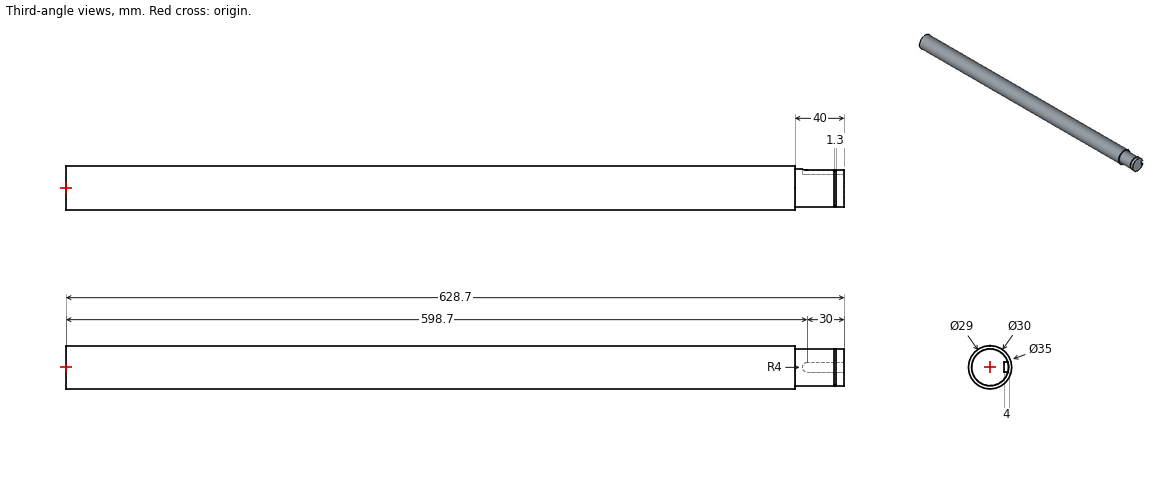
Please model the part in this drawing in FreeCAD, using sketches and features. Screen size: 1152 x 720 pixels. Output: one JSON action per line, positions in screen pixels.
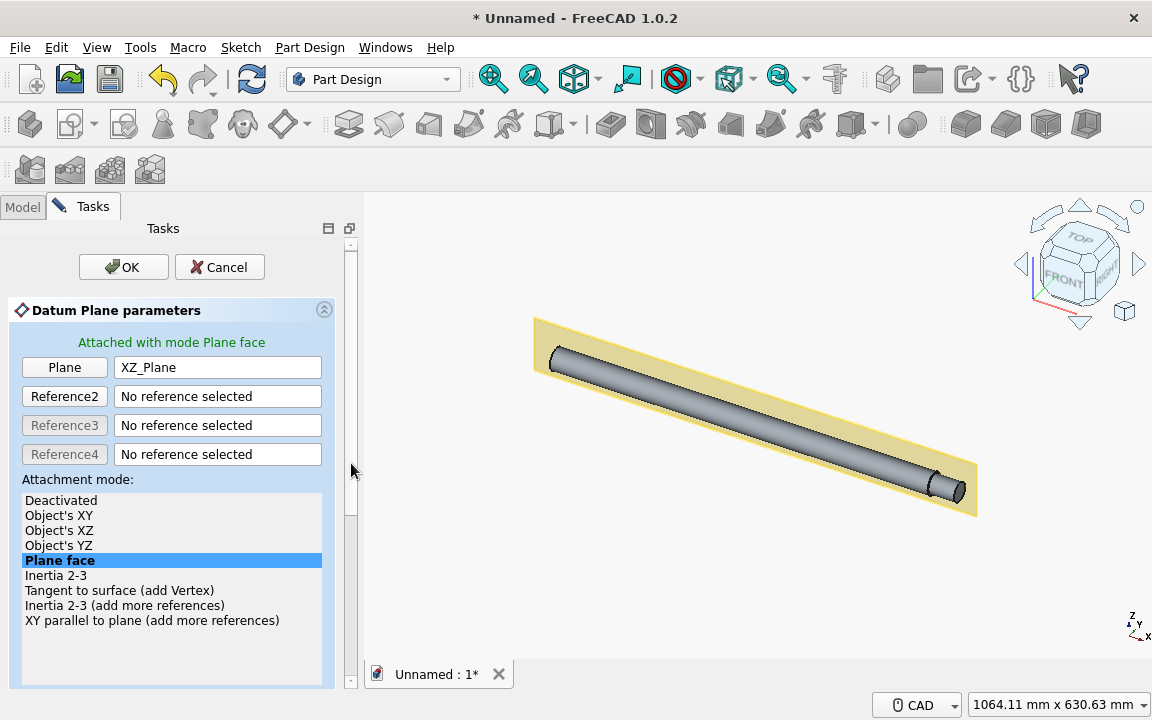
{"action": "left_click", "coordinate": [124, 267]}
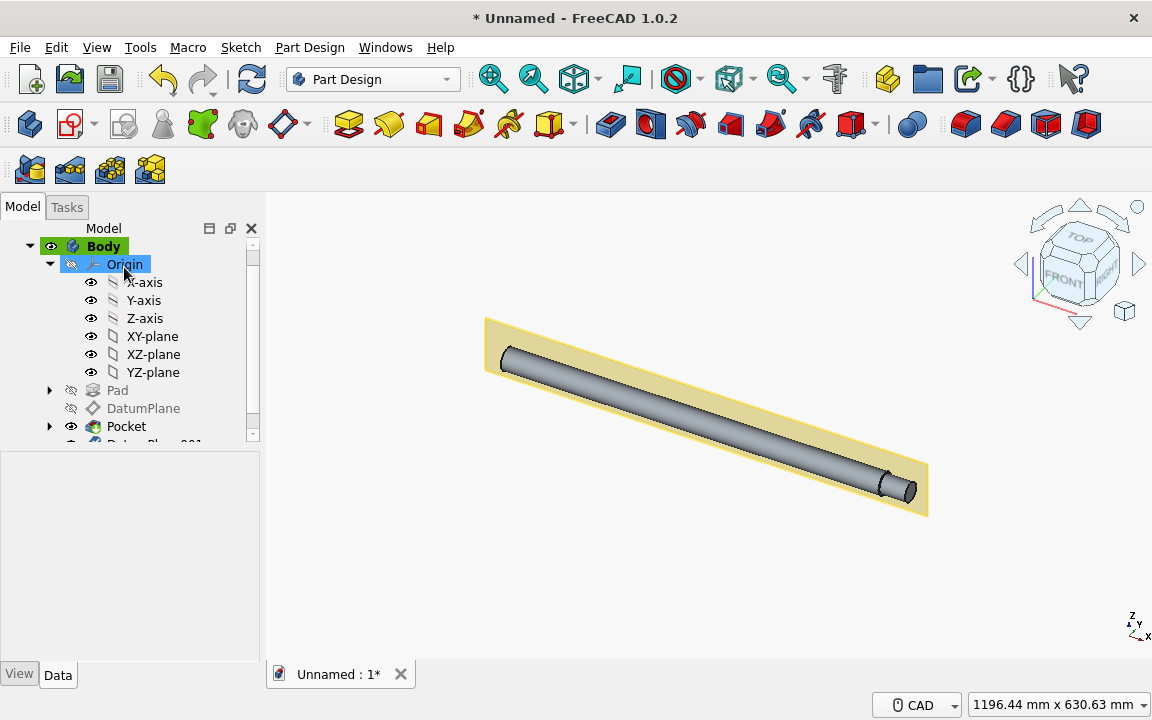
{"action": "scroll", "coordinate": [120, 332], "scroll_direction": "down", "scroll_amount": 3}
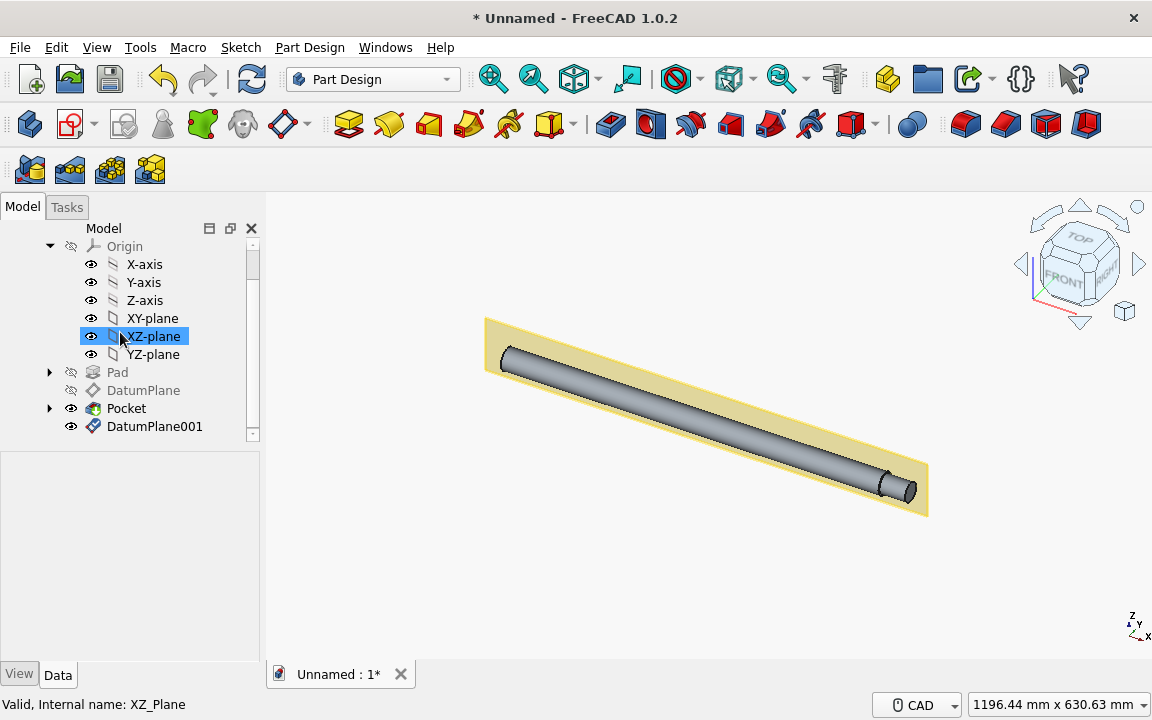
{"action": "left_click", "coordinate": [116, 426]}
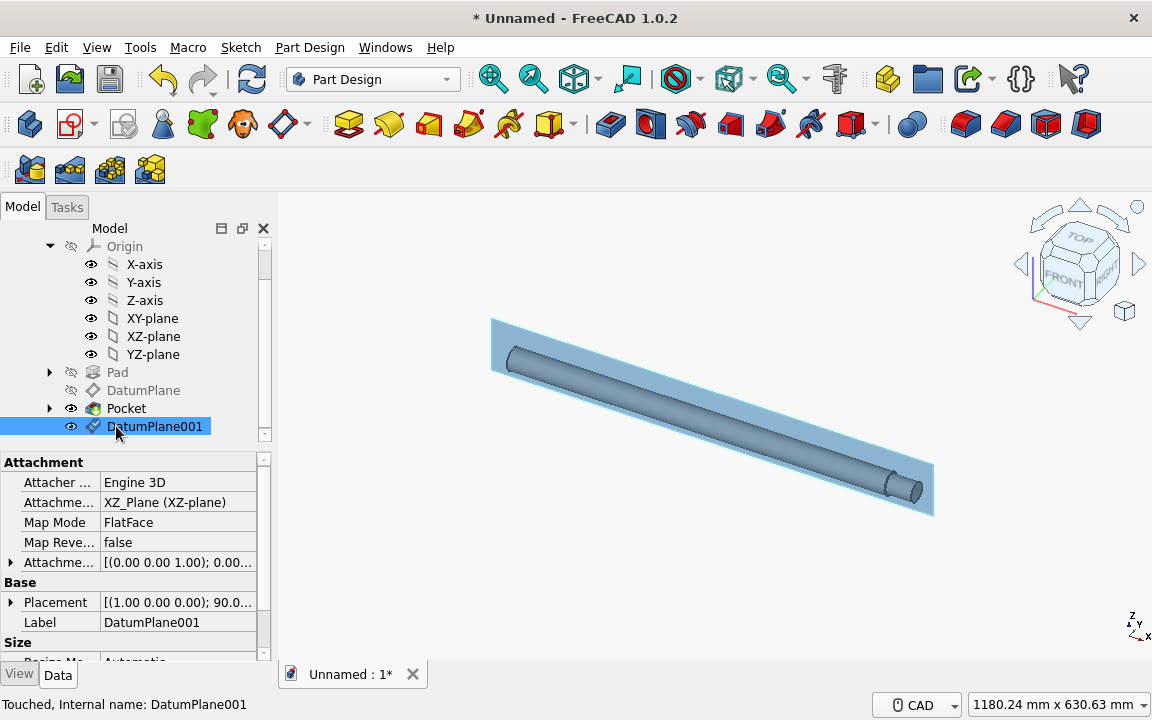
{"action": "left_click", "coordinate": [70, 124]}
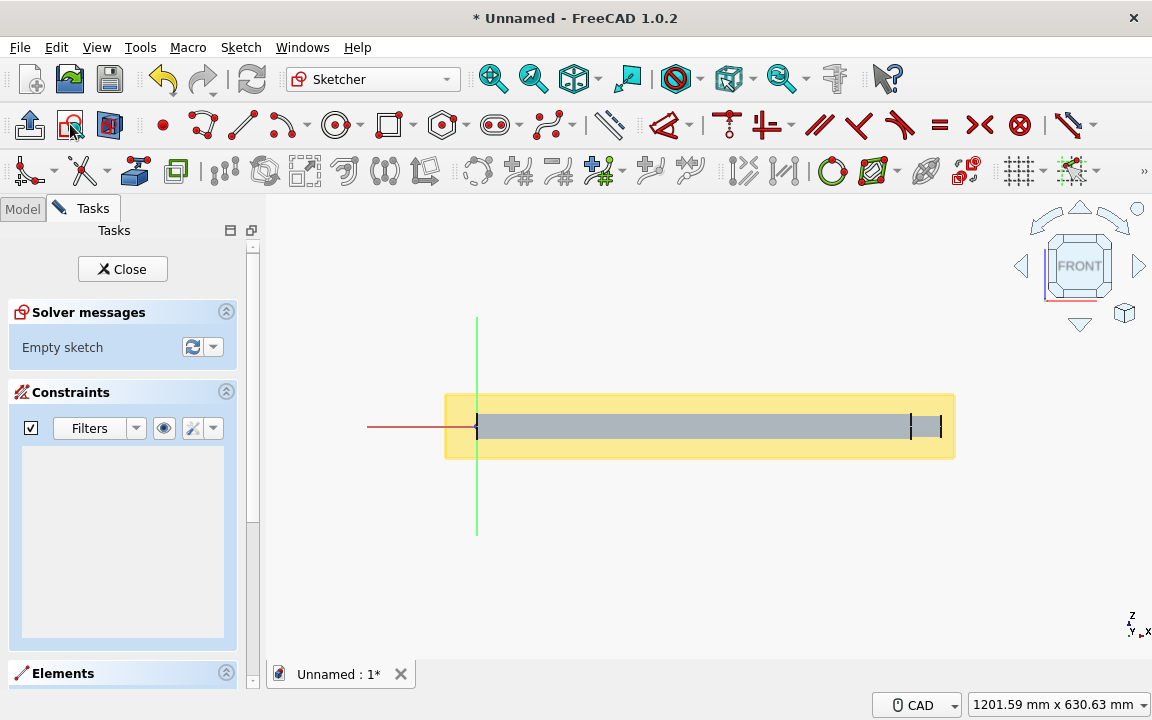
{"action": "left_click", "coordinate": [110, 126]}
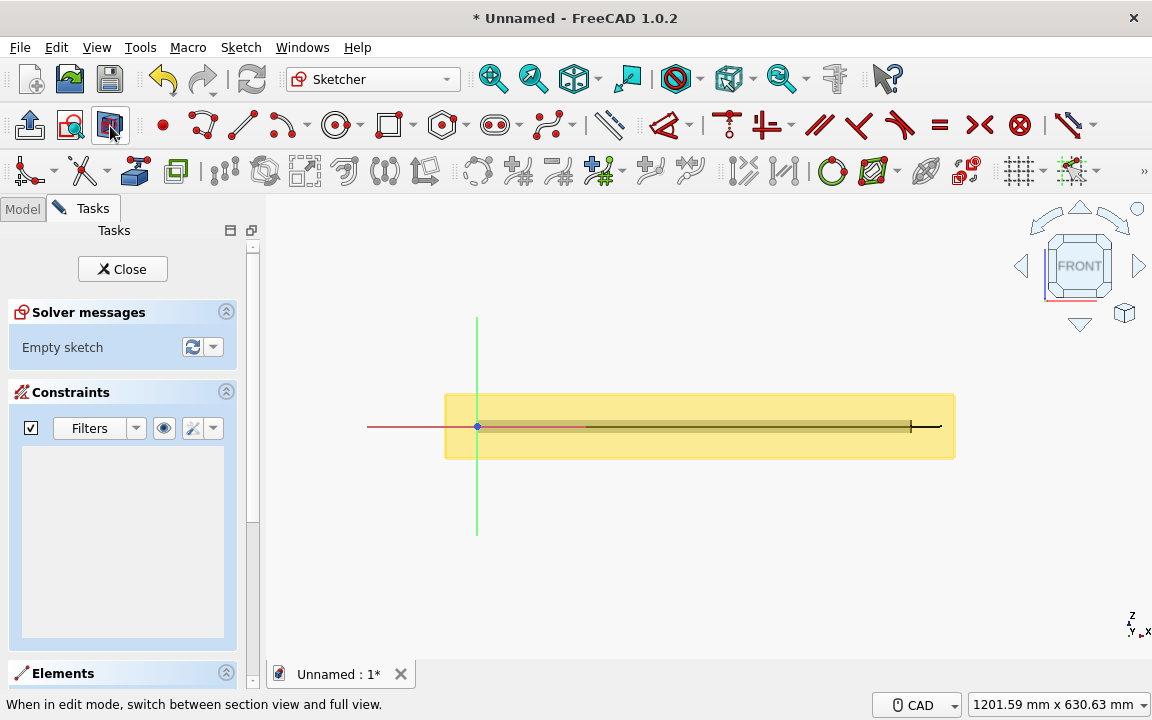
{"action": "scroll", "coordinate": [943, 426], "scroll_direction": "up", "scroll_amount": 15}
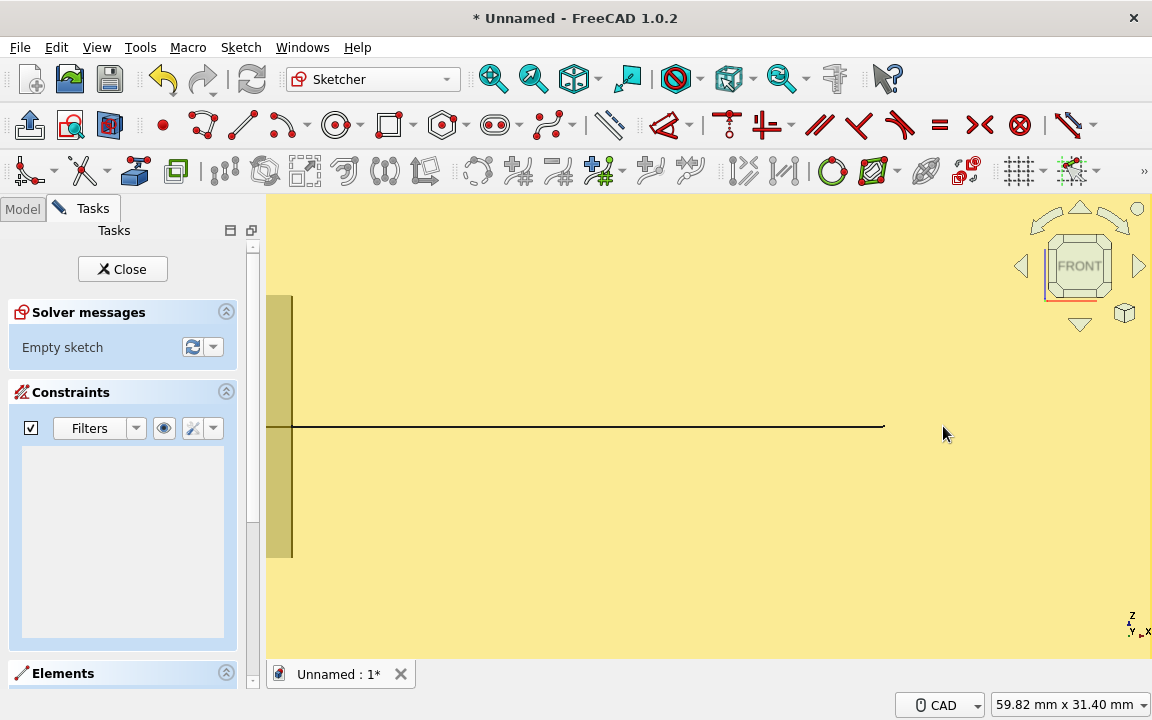
{"action": "left_click", "coordinate": [204, 126]}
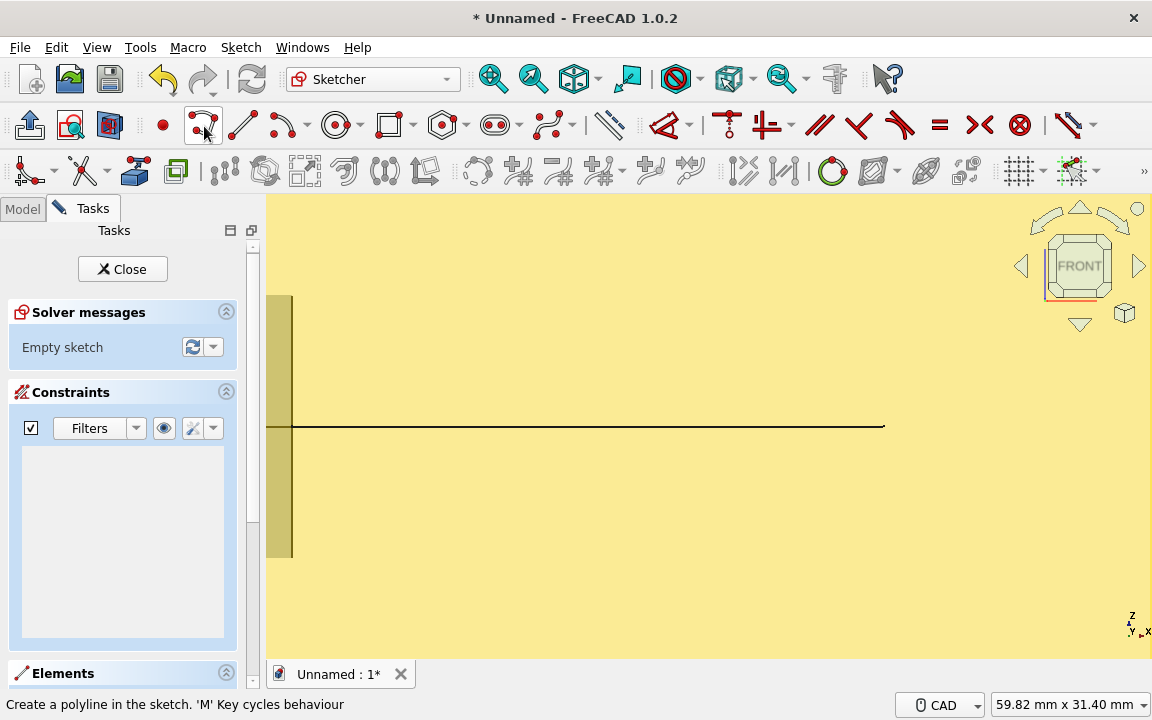
{"action": "left_click", "coordinate": [440, 367]}
{"action": "left_click", "coordinate": [884, 367]}
{"action": "left_click", "coordinate": [884, 486]}
{"action": "left_click", "coordinate": [440, 486]}
{"action": "right_click", "coordinate": [440, 486]}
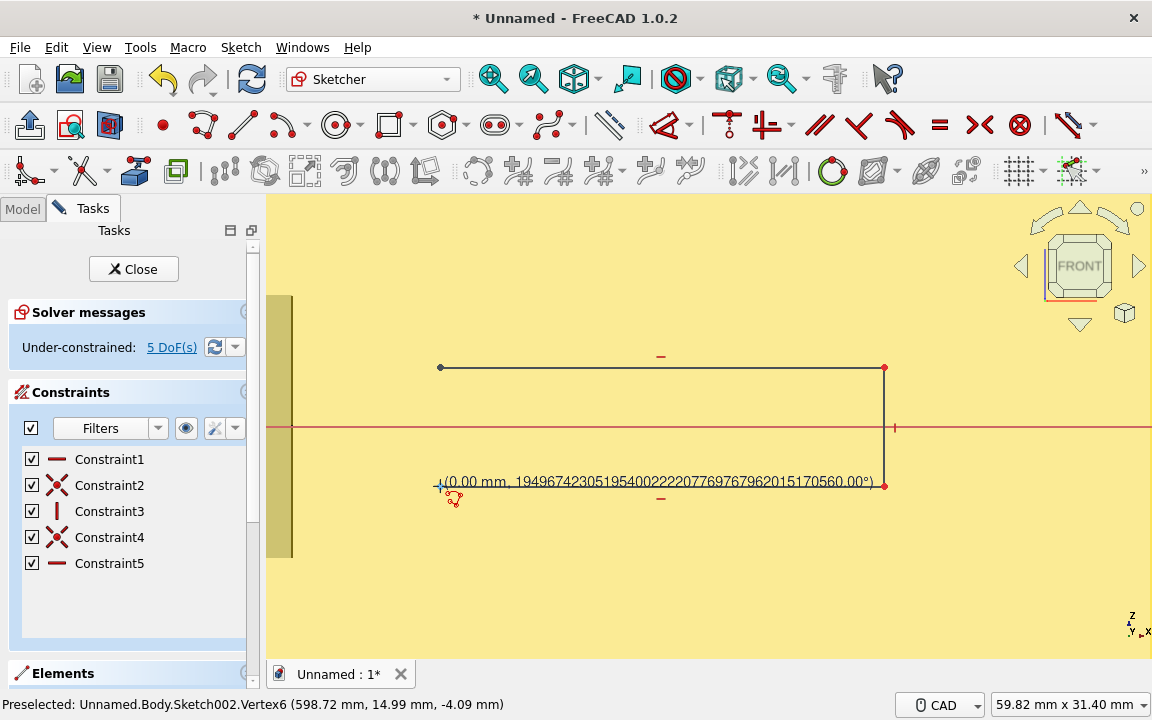
{"action": "left_click", "coordinate": [310, 126]}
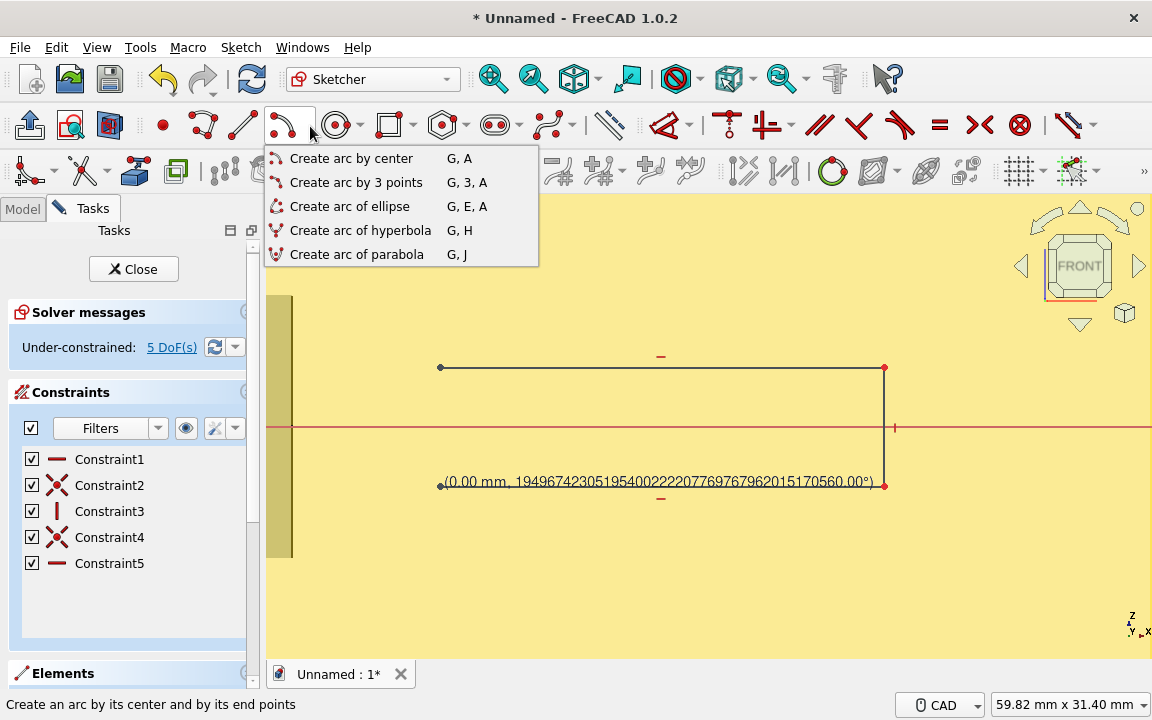
{"action": "left_click", "coordinate": [402, 182]}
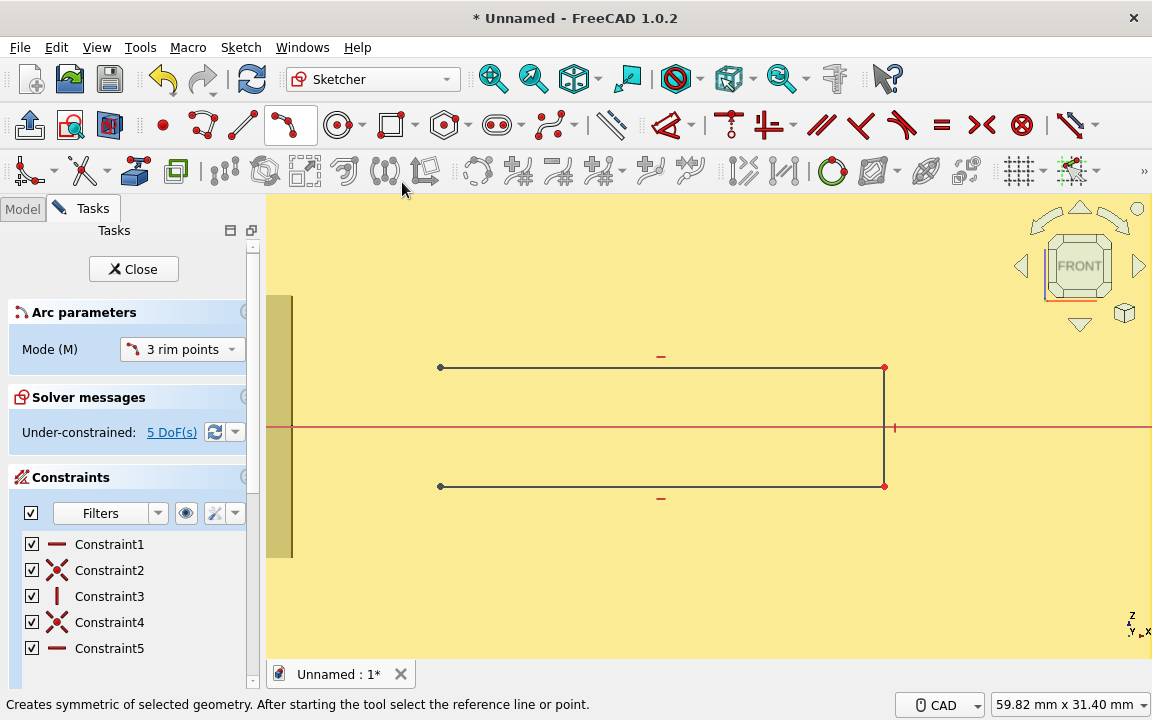
{"action": "left_click", "coordinate": [440, 487]}
{"action": "left_click", "coordinate": [440, 368]}
{"action": "left_click", "coordinate": [383, 408]}
{"action": "key", "text": "Escape"}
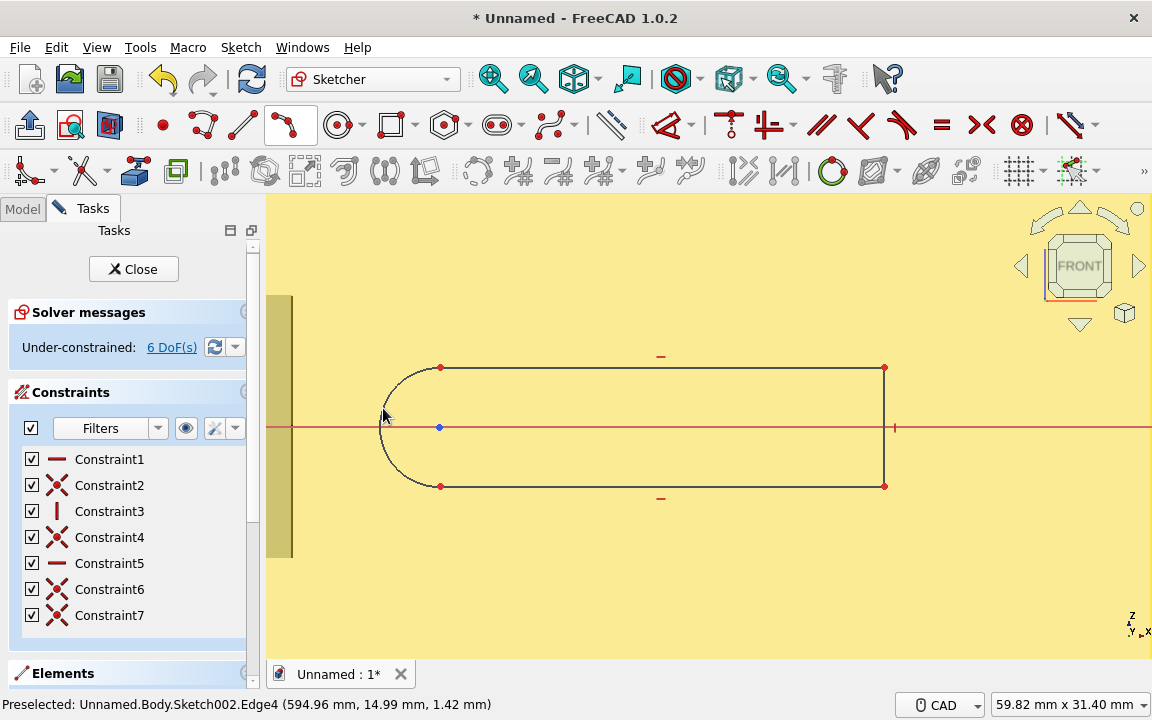
{"action": "left_click", "coordinate": [573, 368]}